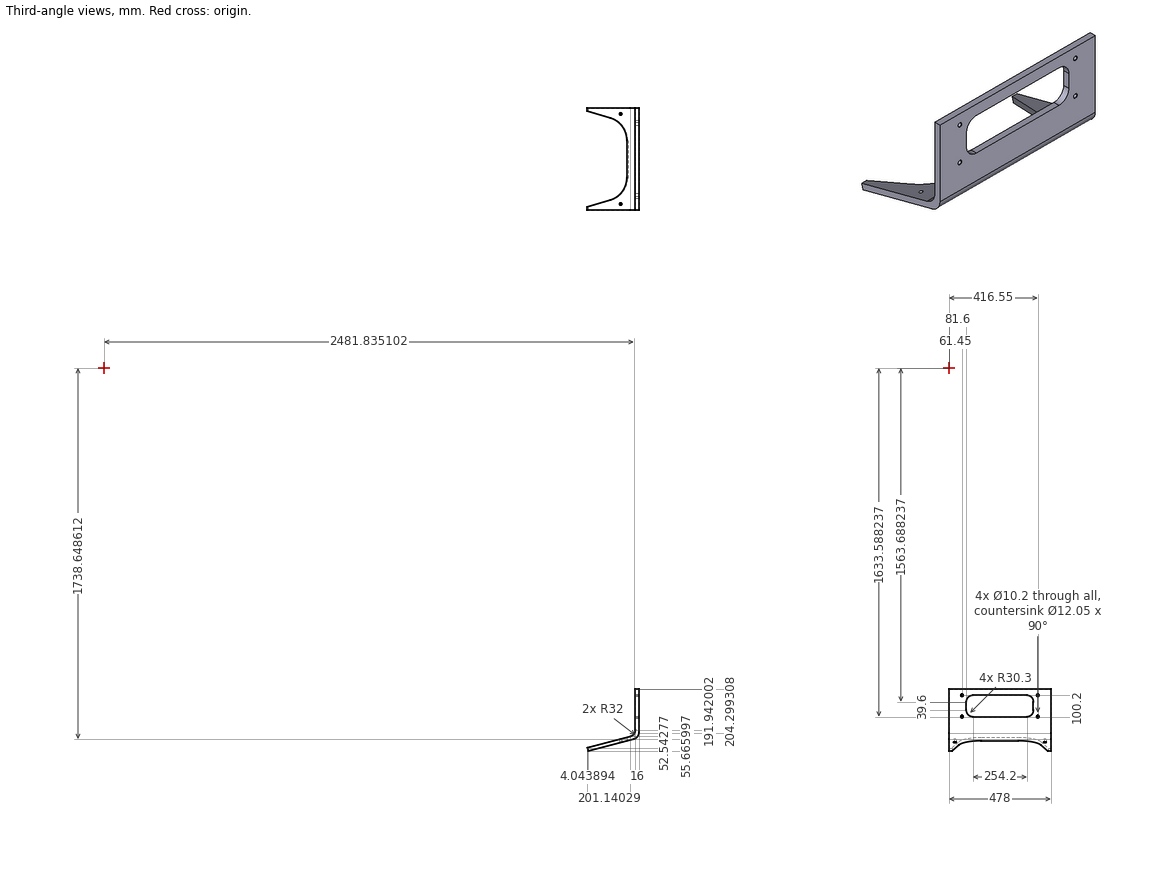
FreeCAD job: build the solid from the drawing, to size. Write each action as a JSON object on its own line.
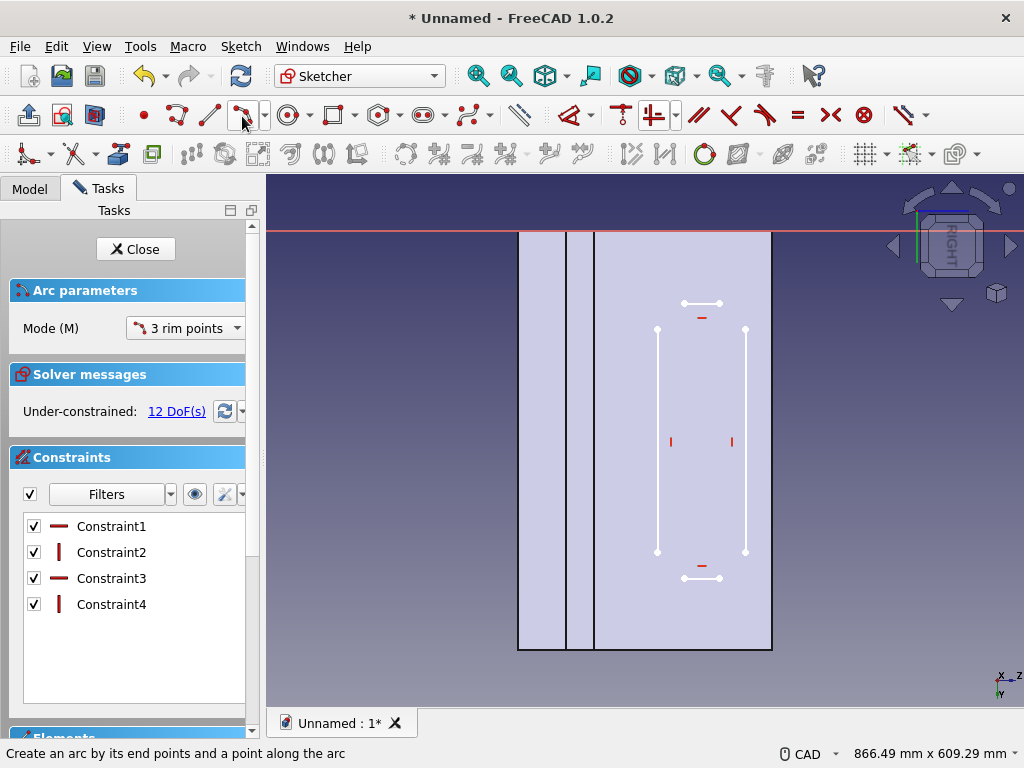
{"action": "left_click", "coordinate": [685, 304]}
{"action": "left_click", "coordinate": [658, 330]}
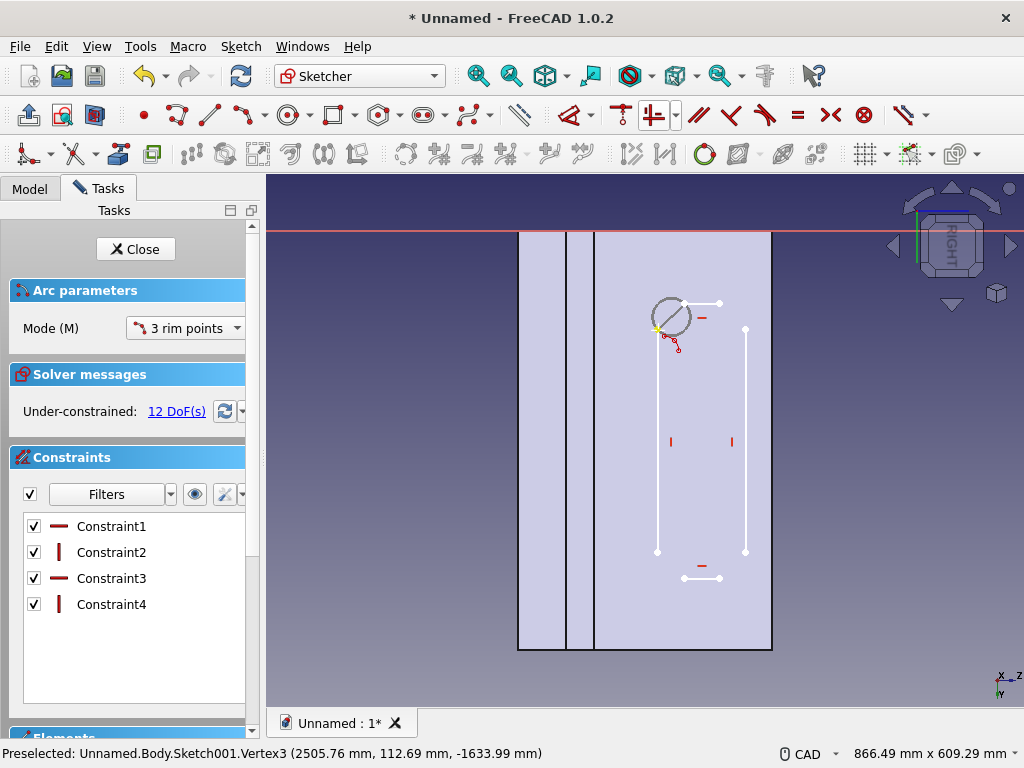
{"action": "scroll", "coordinate": [666, 311], "scroll_direction": "up", "scroll_amount": 4}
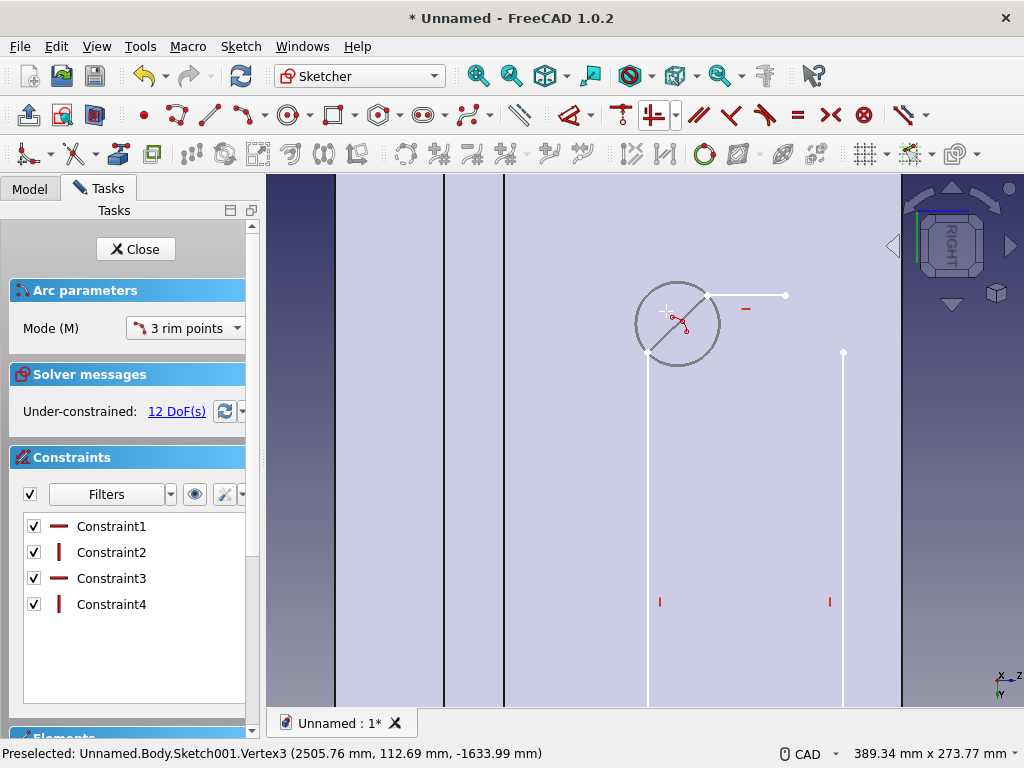
{"action": "left_click", "coordinate": [666, 310]}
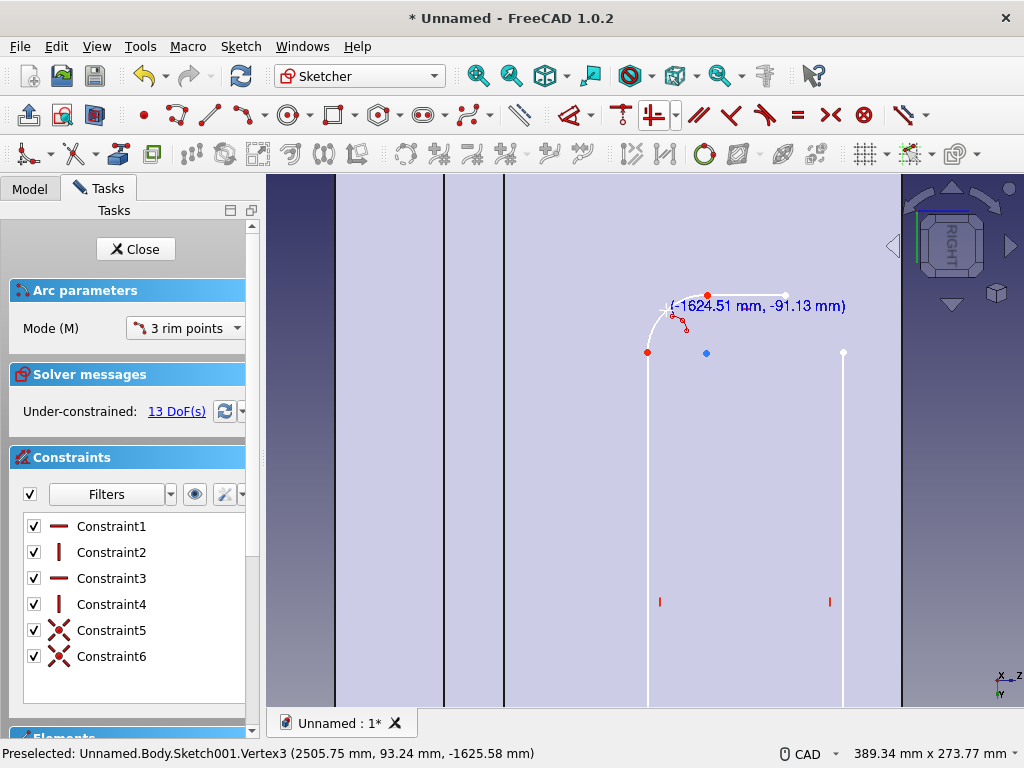
{"action": "scroll", "coordinate": [370, 248], "scroll_direction": "down", "scroll_amount": 3}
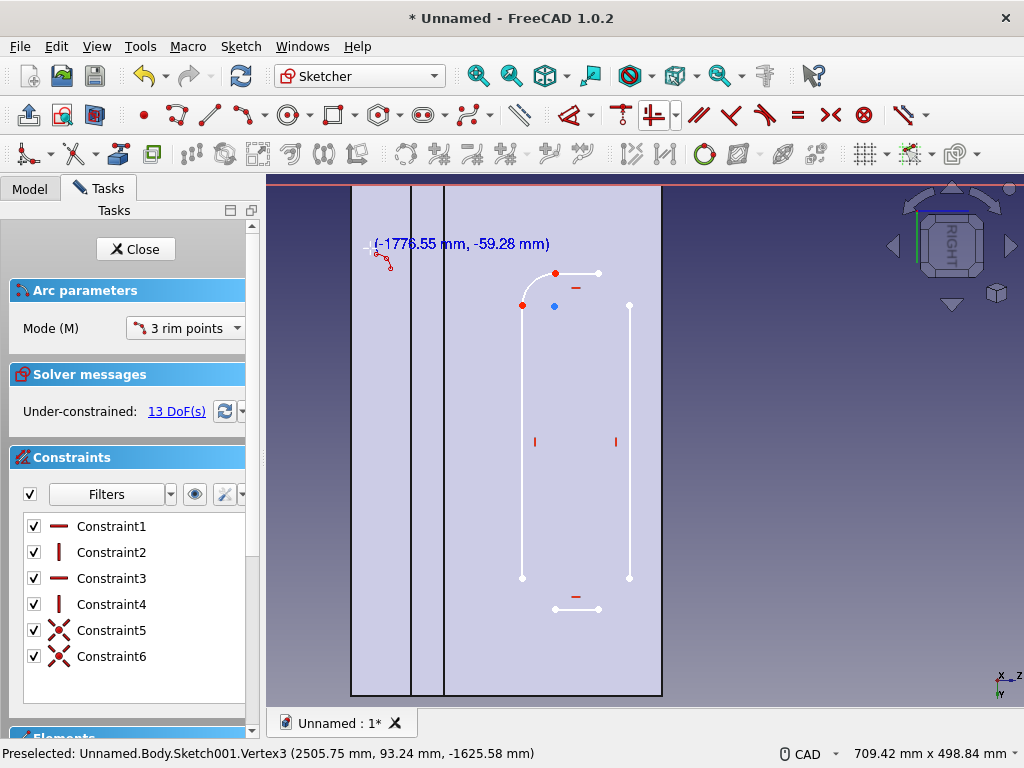
{"action": "left_click", "coordinate": [522, 578]}
{"action": "left_click", "coordinate": [555, 610]}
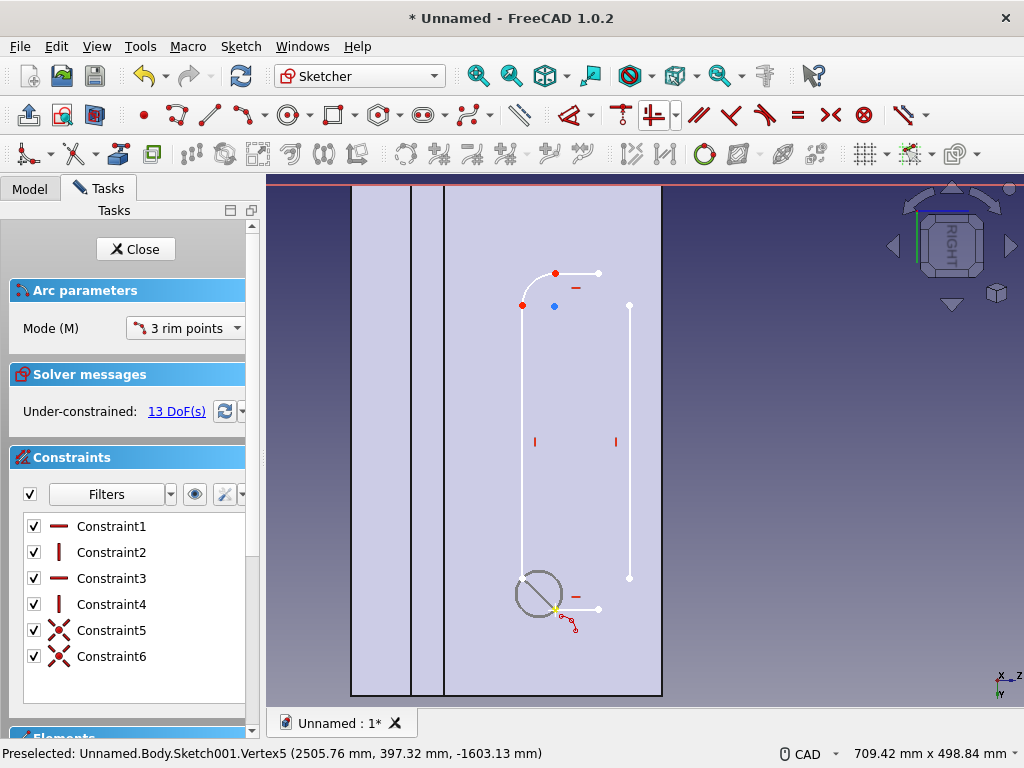
{"action": "scroll", "coordinate": [532, 599], "scroll_direction": "up", "scroll_amount": 3}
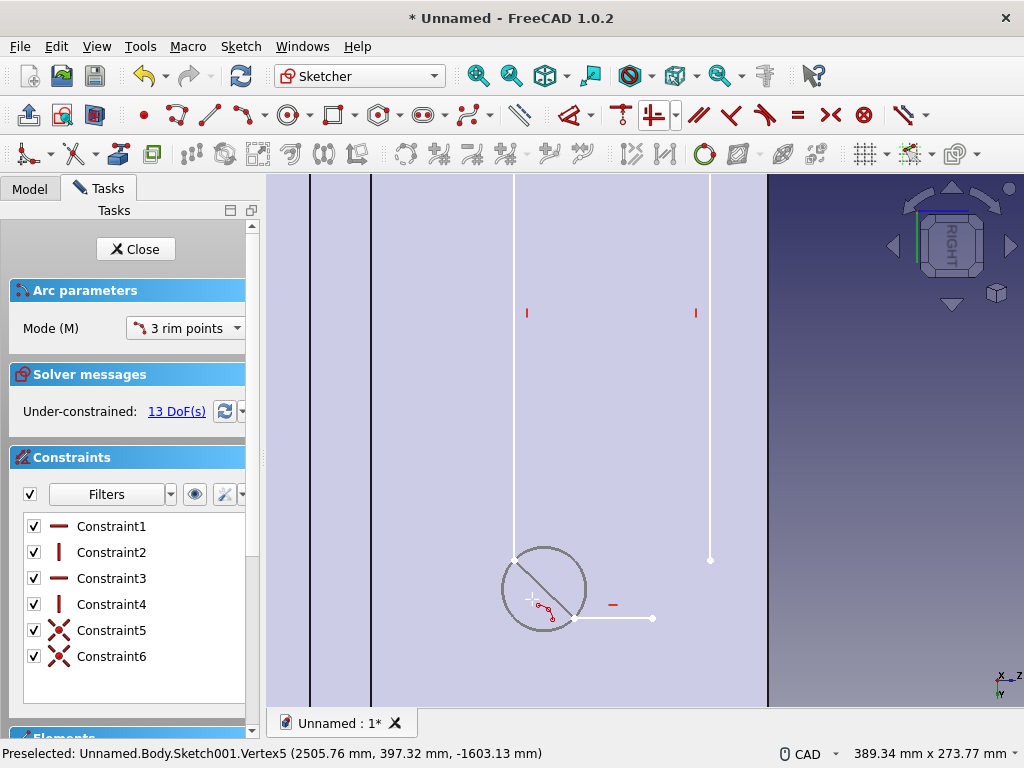
{"action": "left_click", "coordinate": [532, 599]}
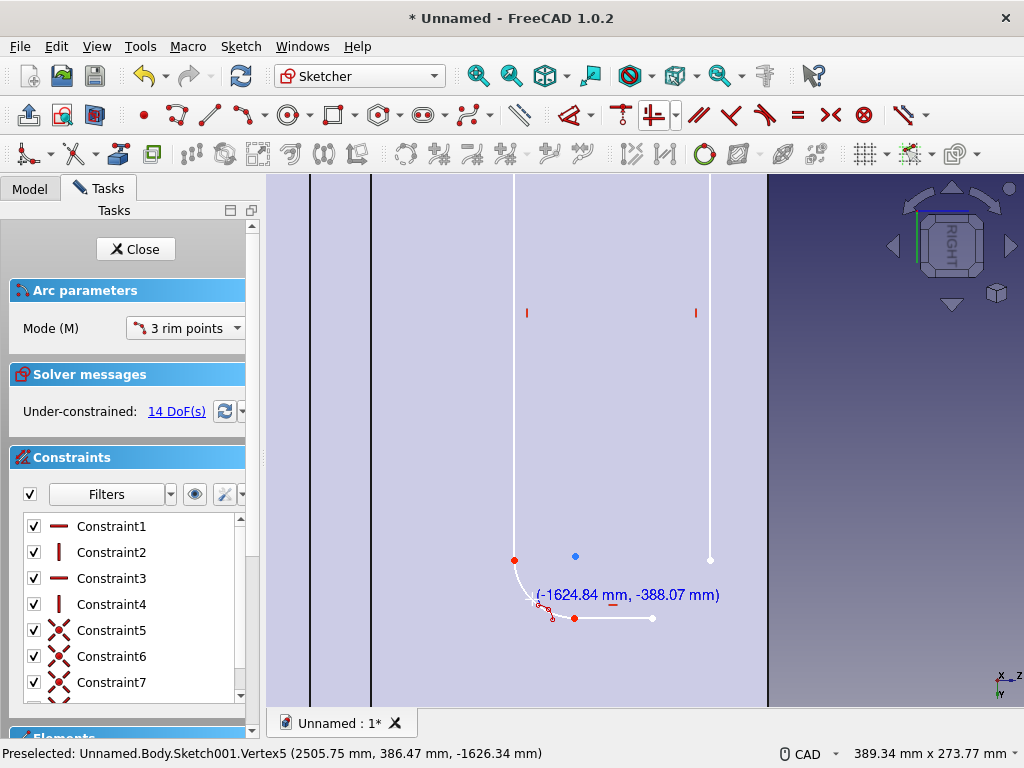
{"action": "left_click", "coordinate": [652, 618]}
{"action": "left_click", "coordinate": [710, 560]}
{"action": "left_click", "coordinate": [693, 599]}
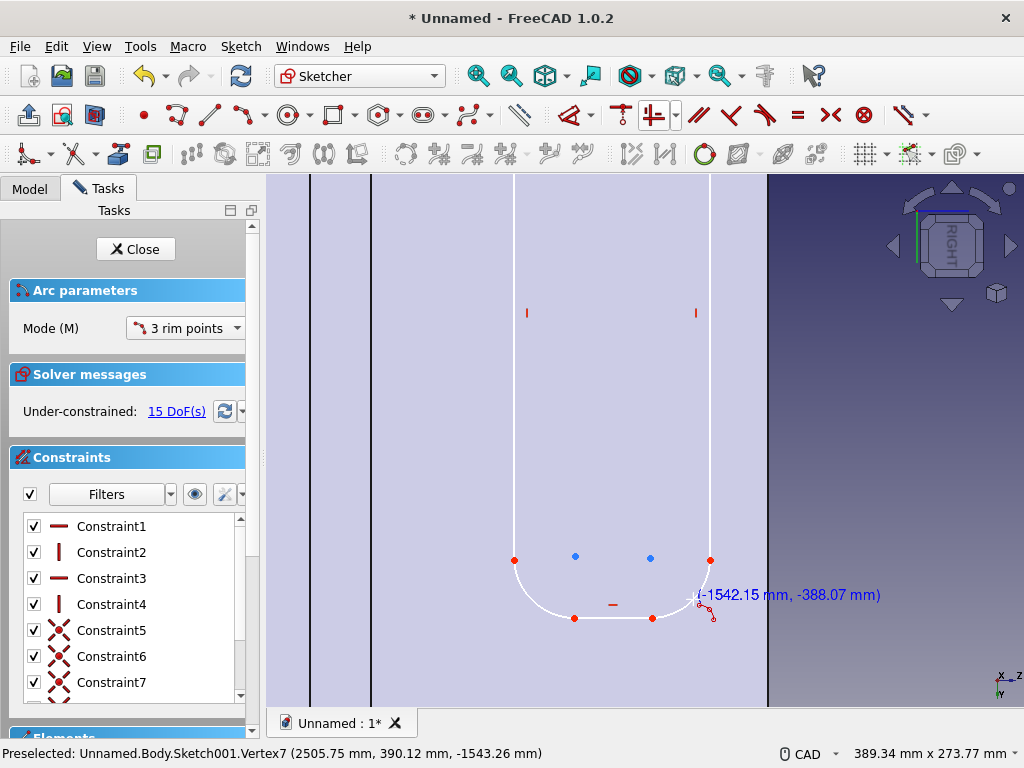
{"action": "scroll", "coordinate": [533, 599], "scroll_direction": "down", "scroll_amount": 3}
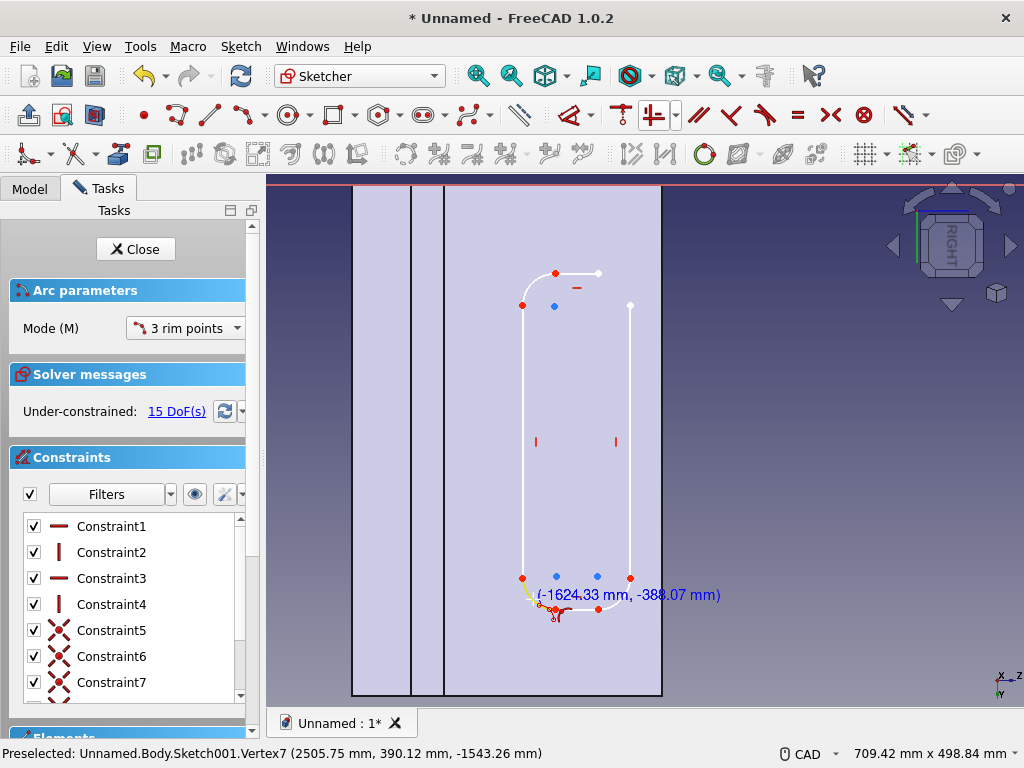
{"action": "left_click", "coordinate": [630, 306]}
{"action": "left_click", "coordinate": [599, 274]}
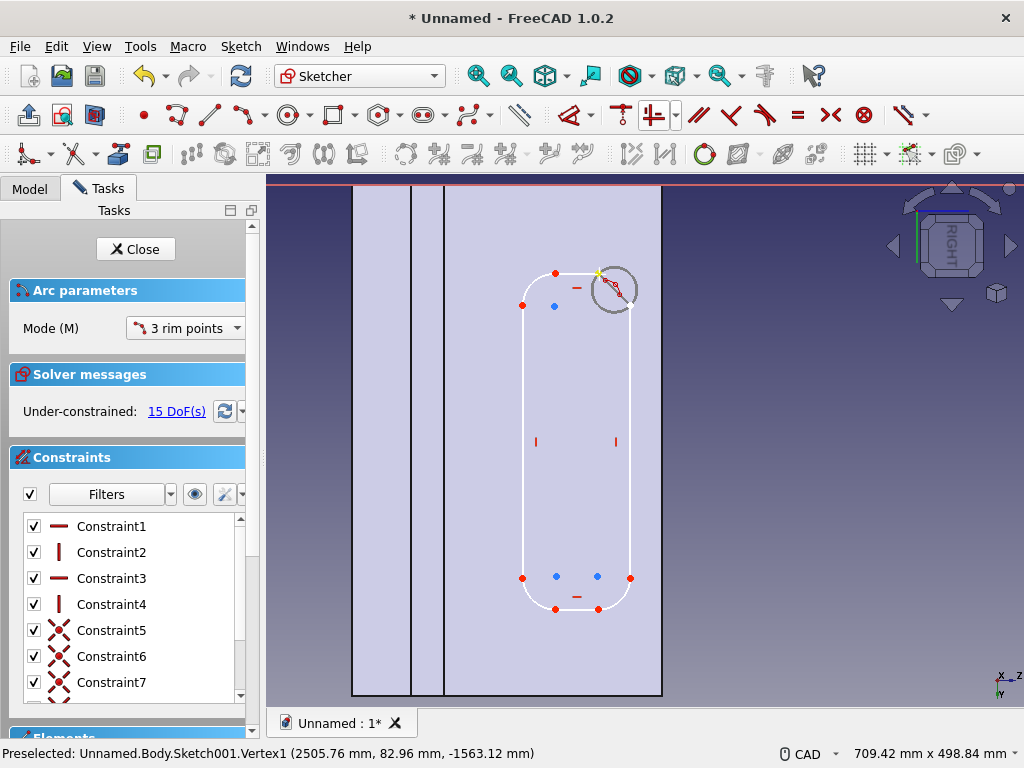
{"action": "scroll", "coordinate": [621, 282], "scroll_direction": "up", "scroll_amount": 3}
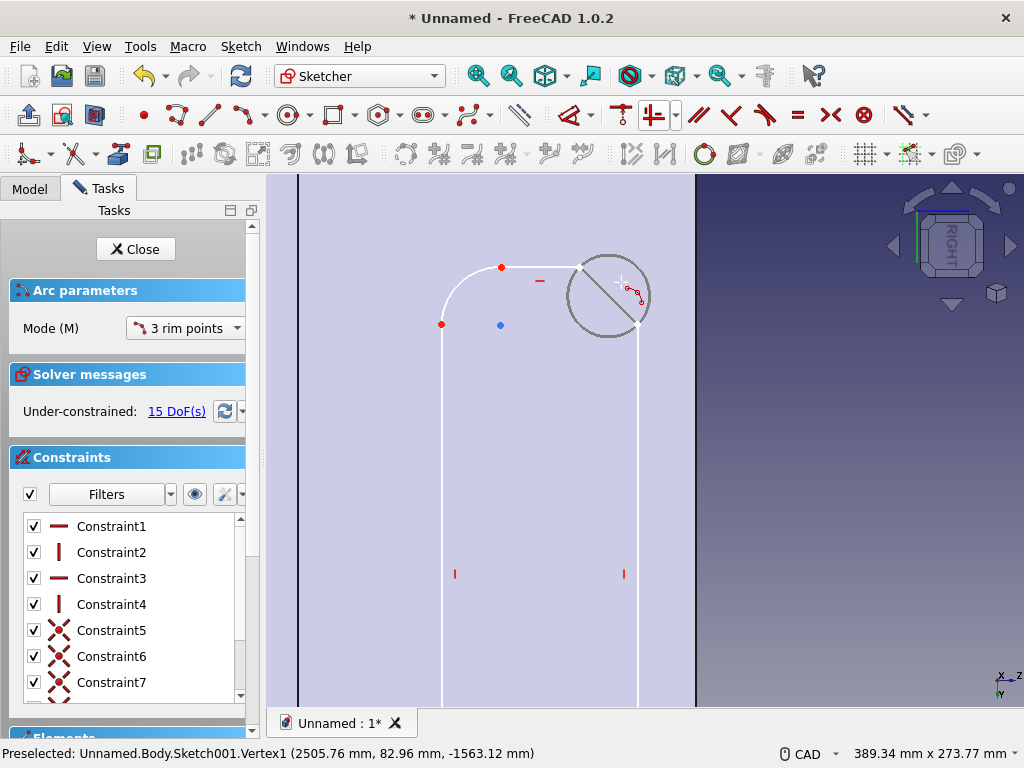
{"action": "left_click", "coordinate": [620, 282]}
{"action": "key", "text": "Escape"}